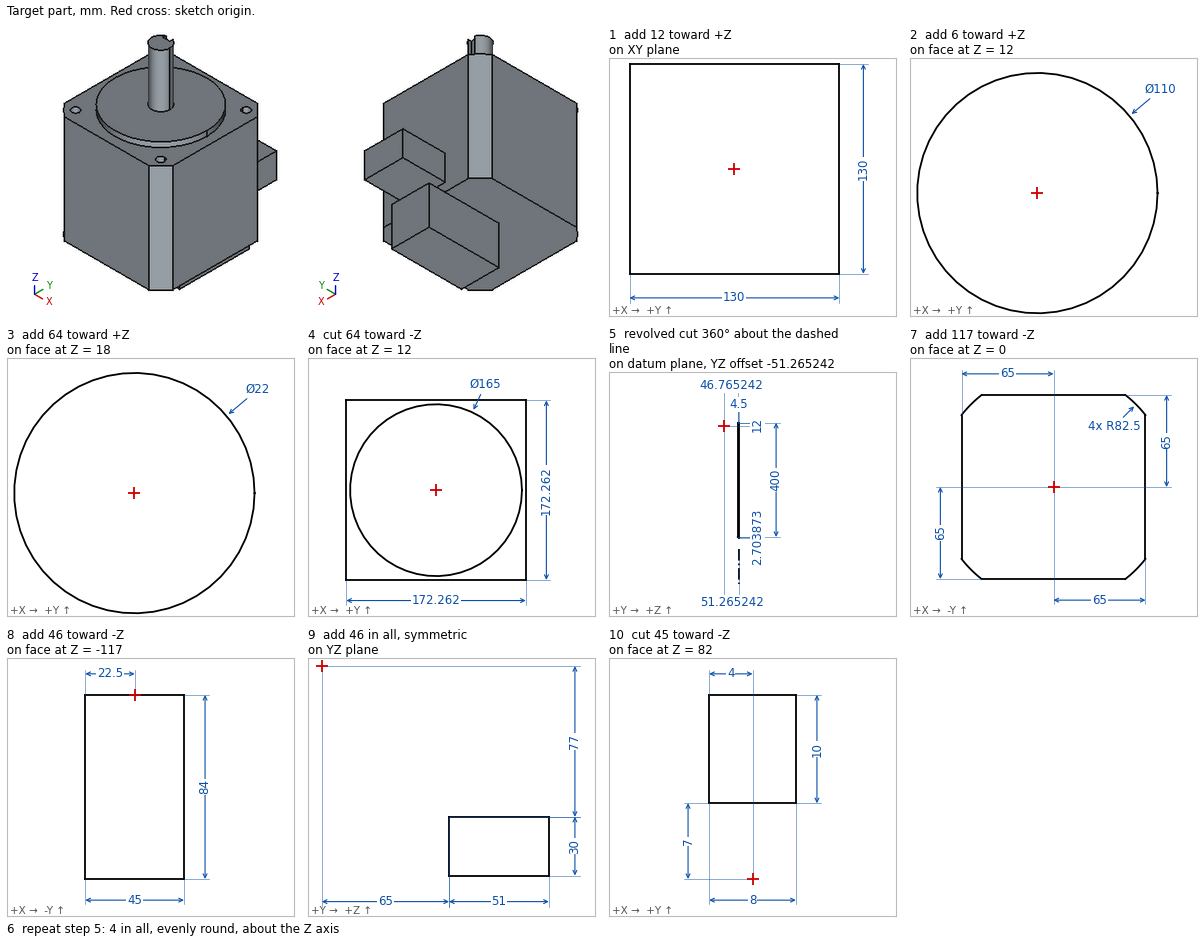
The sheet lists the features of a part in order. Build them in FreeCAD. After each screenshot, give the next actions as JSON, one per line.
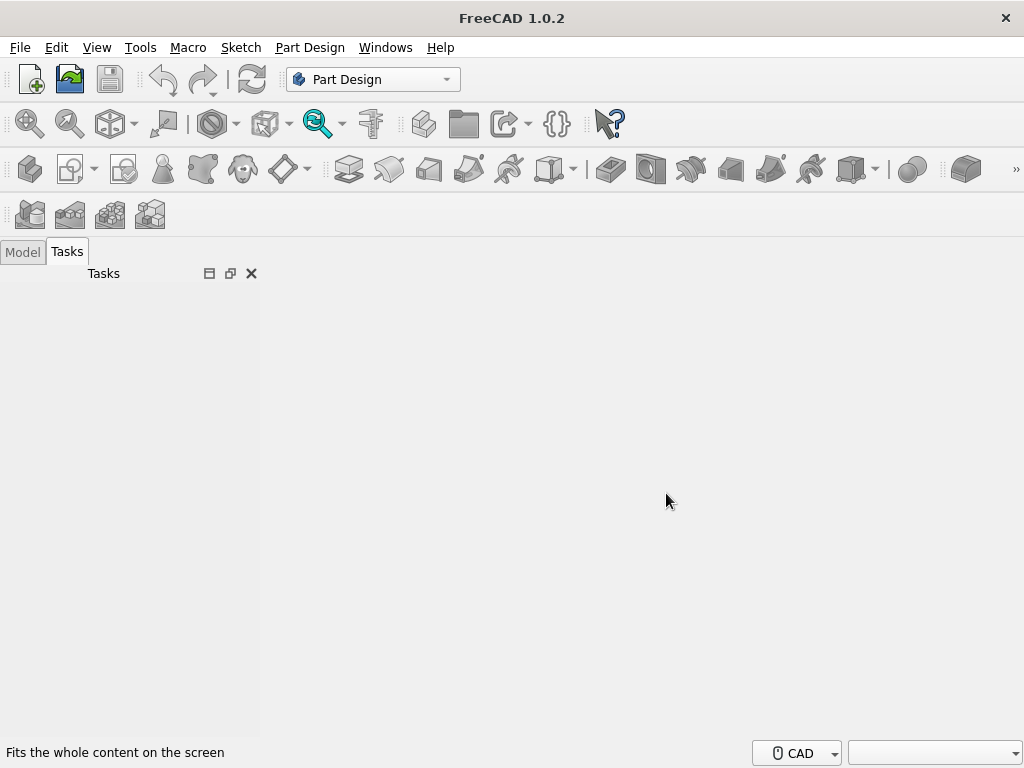
{"action": "left_click", "coordinate": [30, 80]}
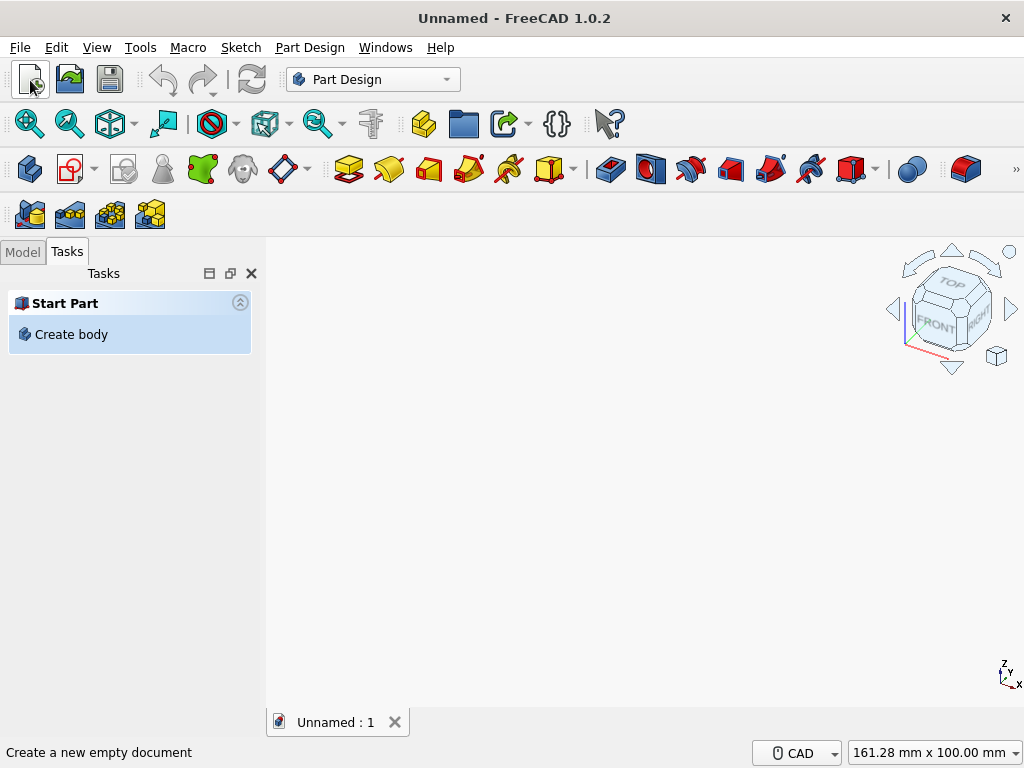
{"action": "left_click", "coordinate": [70, 170]}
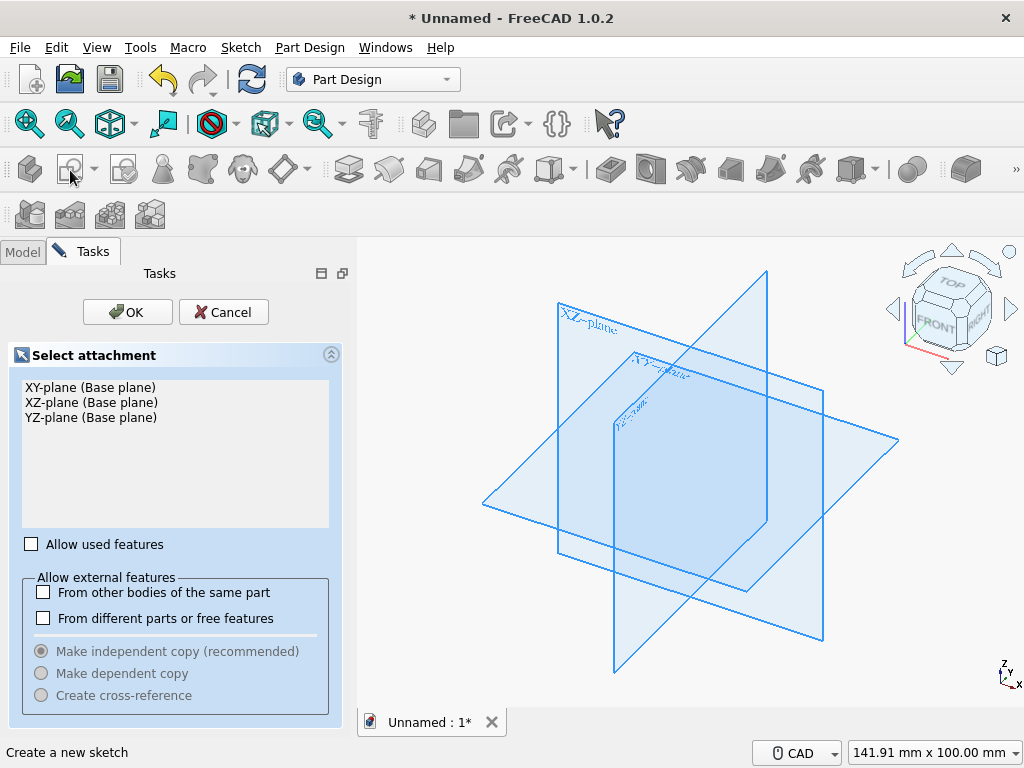
{"action": "left_click", "coordinate": [82, 388]}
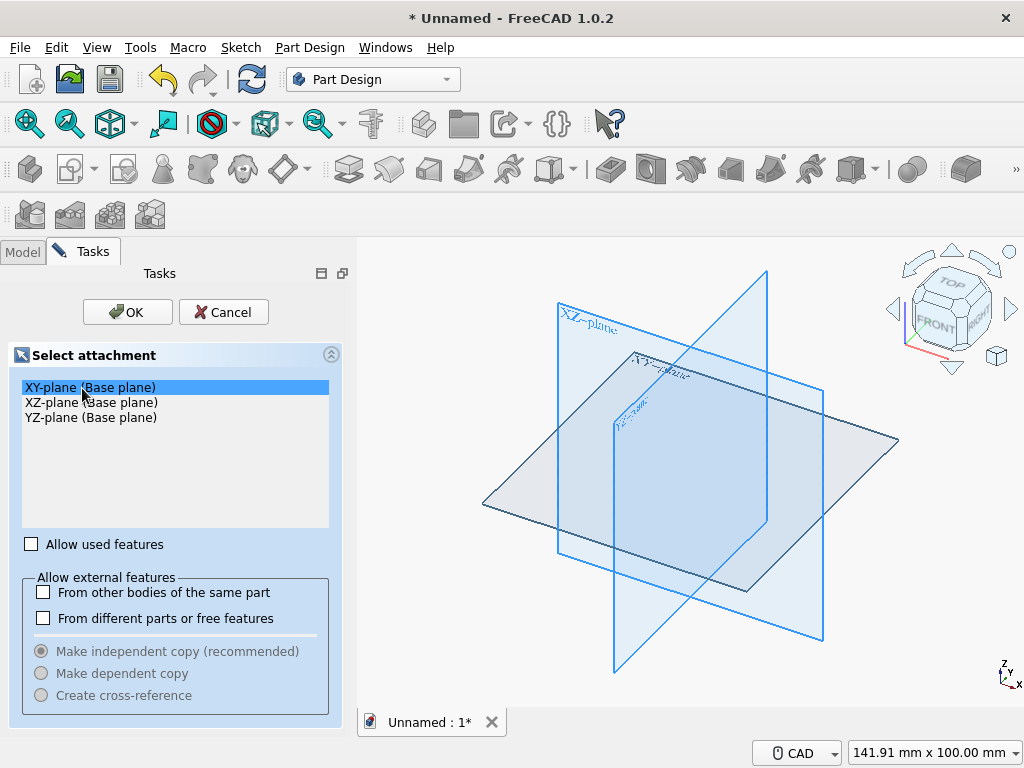
{"action": "left_click", "coordinate": [128, 312]}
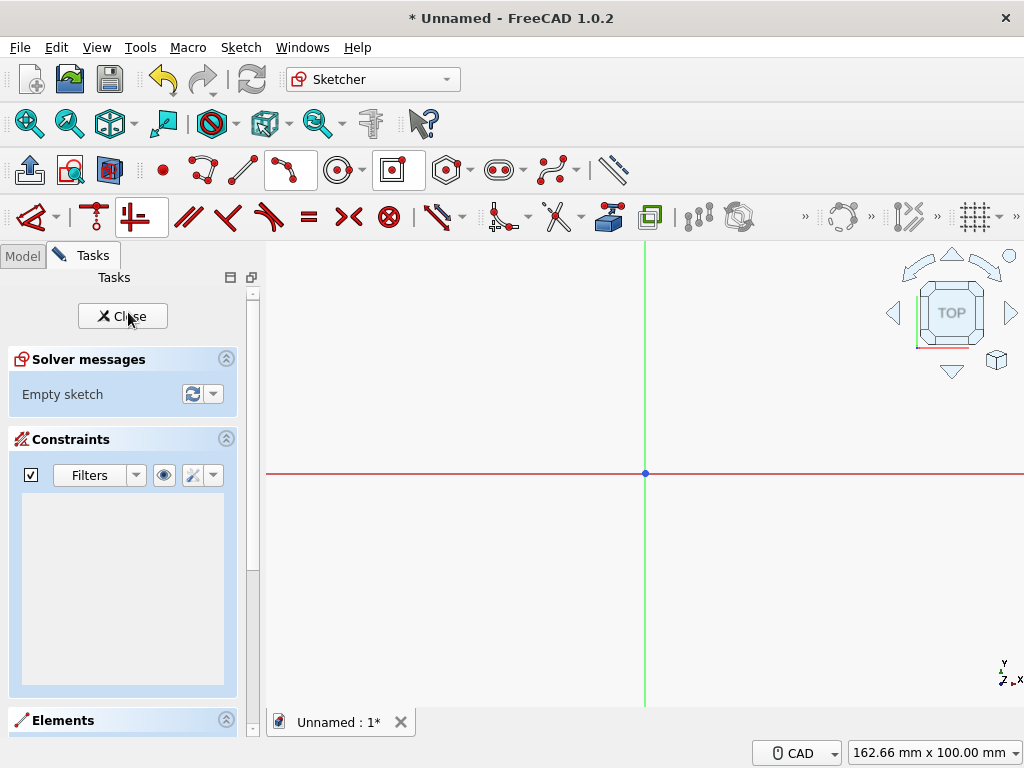
{"action": "scroll", "coordinate": [521, 474], "scroll_direction": "down", "scroll_amount": 4}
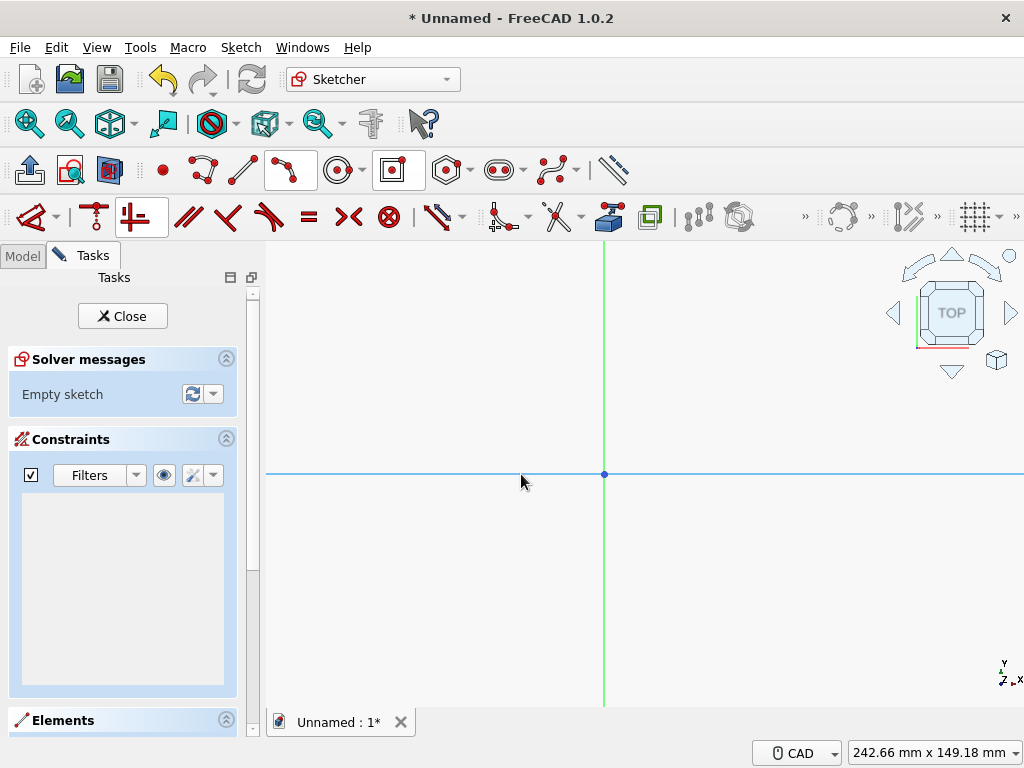
{"action": "left_click", "coordinate": [392, 170]}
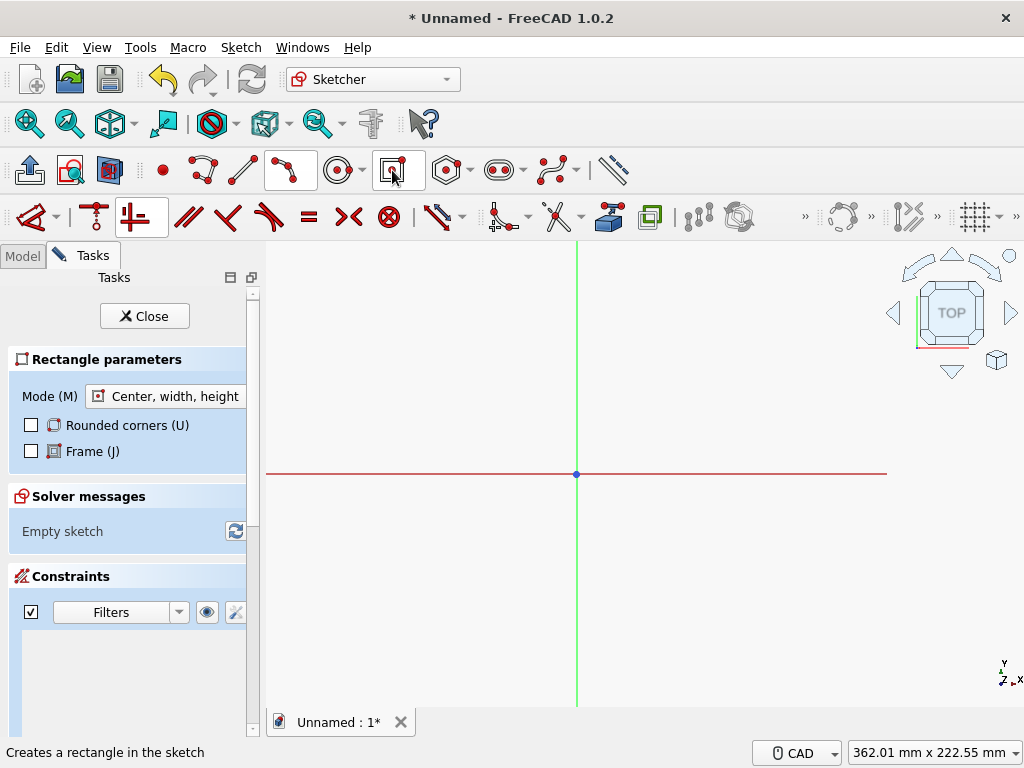
{"action": "left_click", "coordinate": [577, 474]}
{"action": "mouse_move", "coordinate": [713, 338]}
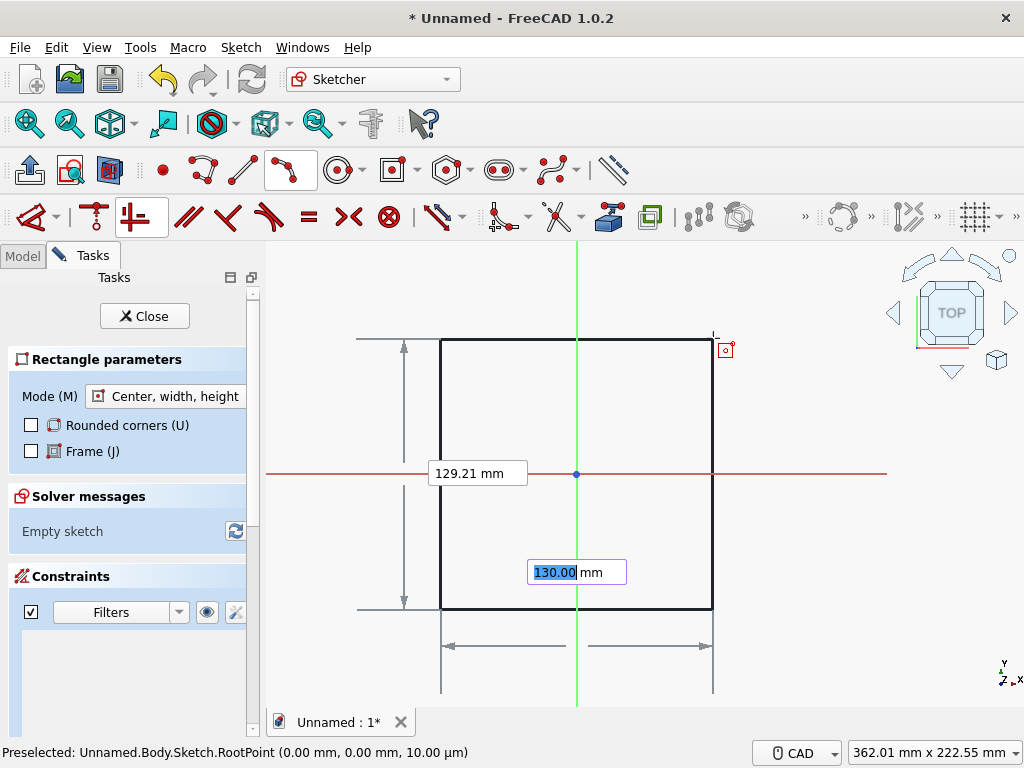
{"action": "type", "text": "130"}
{"action": "key", "text": "Tab"}
{"action": "type", "text": "130"}
{"action": "key", "text": "Return"}
{"action": "key", "text": "Escape"}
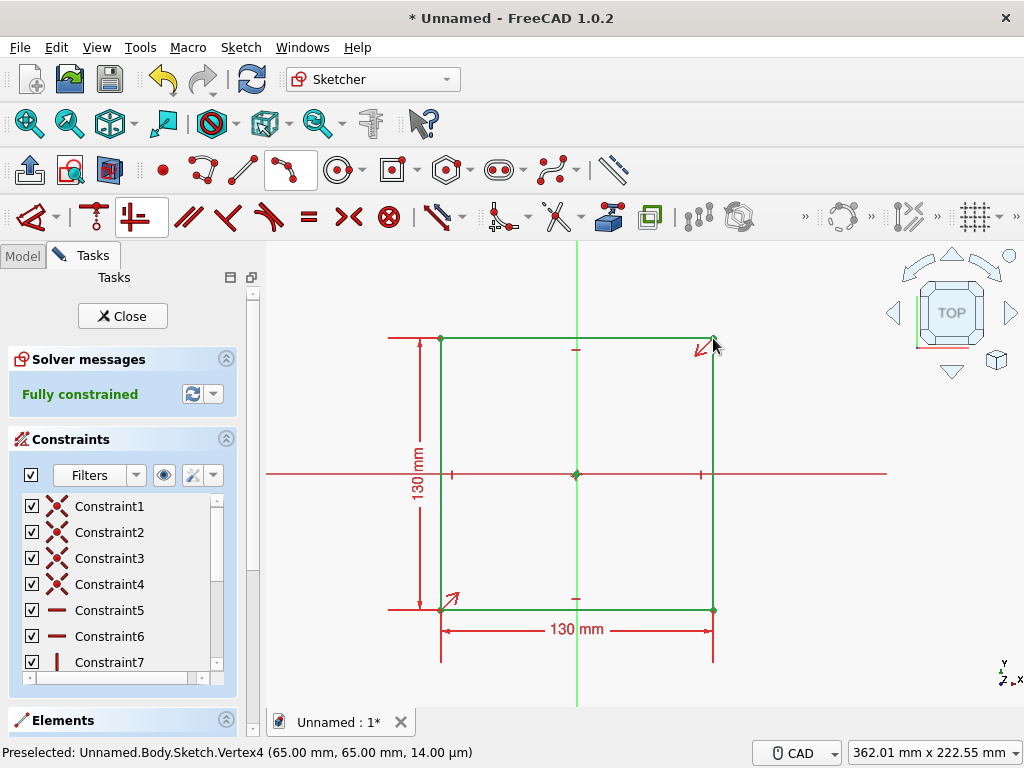
{"action": "left_click", "coordinate": [123, 316]}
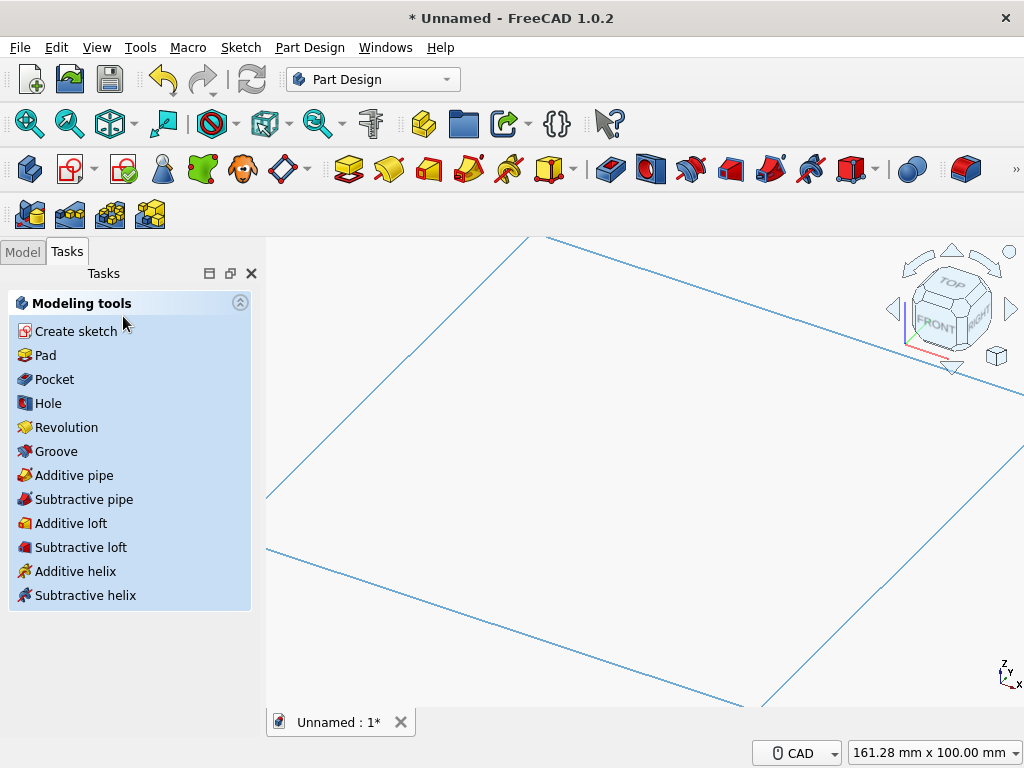
{"action": "left_click", "coordinate": [350, 170]}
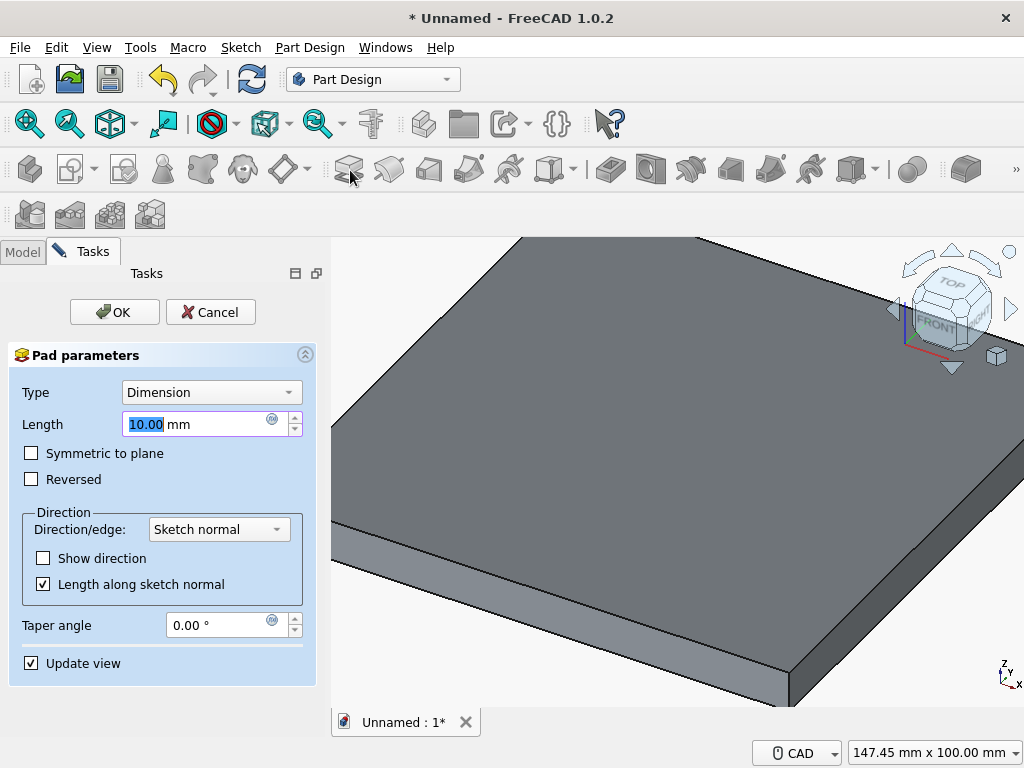
{"action": "type", "text": "12"}
{"action": "key", "text": "Tab"}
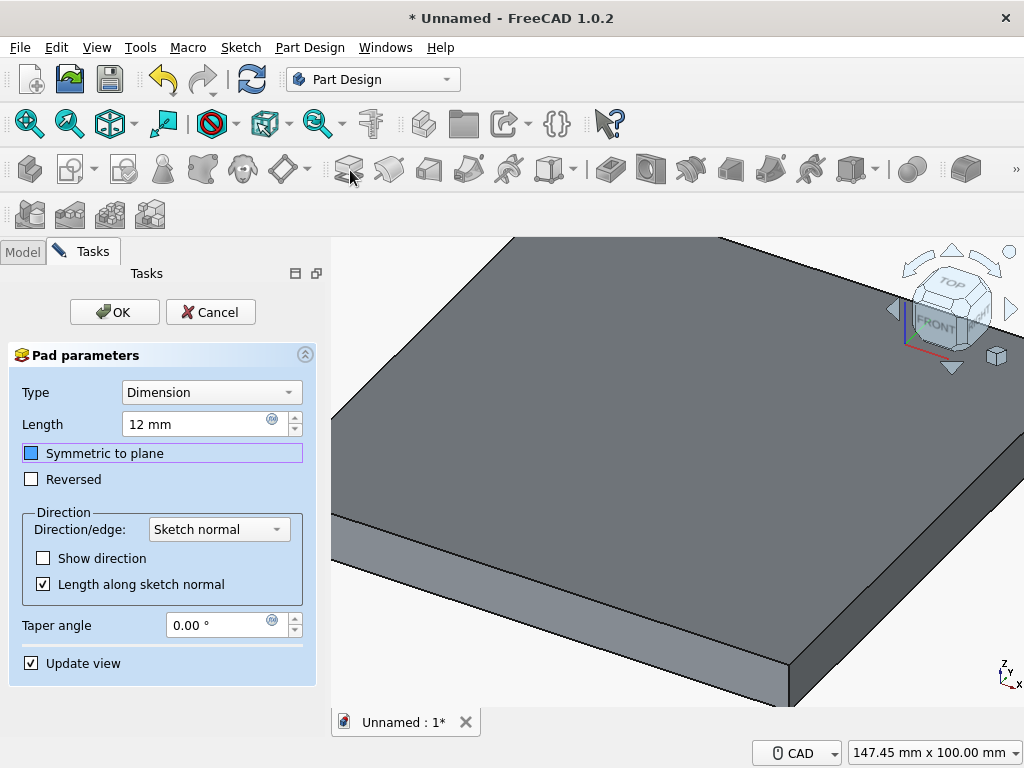
{"action": "left_click", "coordinate": [115, 312]}